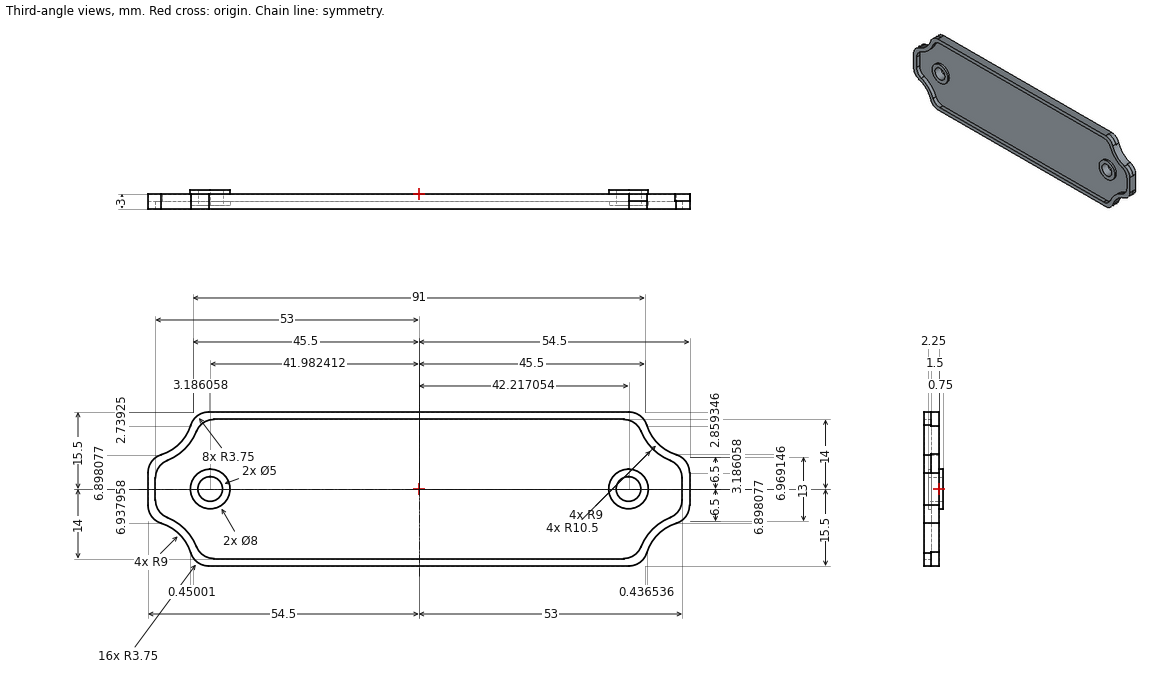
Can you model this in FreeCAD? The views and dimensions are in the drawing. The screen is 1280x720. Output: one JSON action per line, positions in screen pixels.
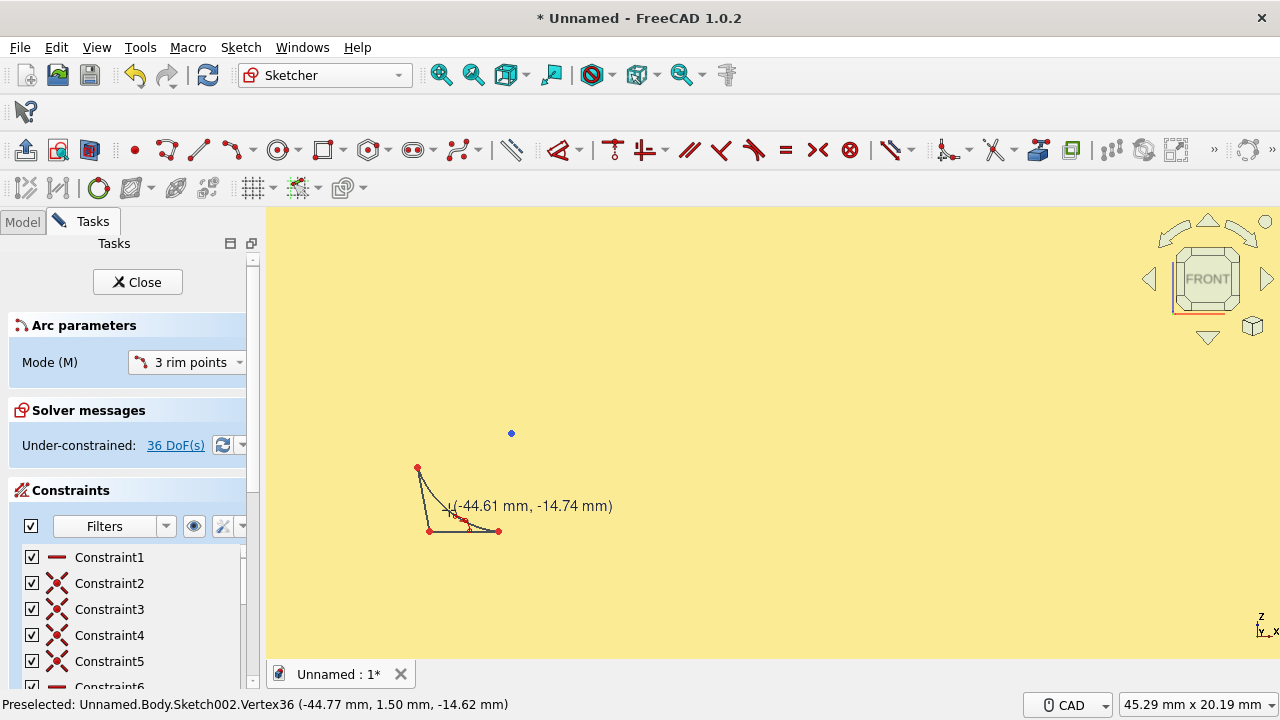
{"action": "left_click", "coordinate": [168, 150]}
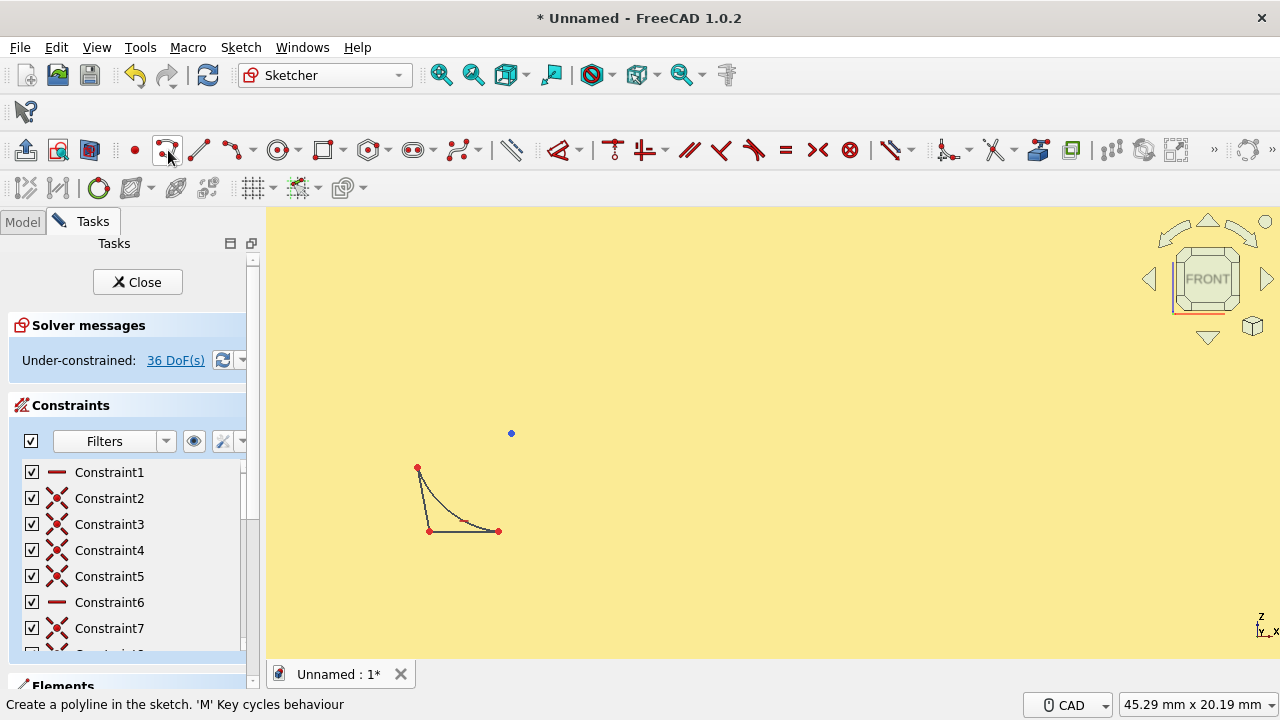
{"action": "scroll", "coordinate": [461, 516], "scroll_direction": "down", "scroll_amount": 7}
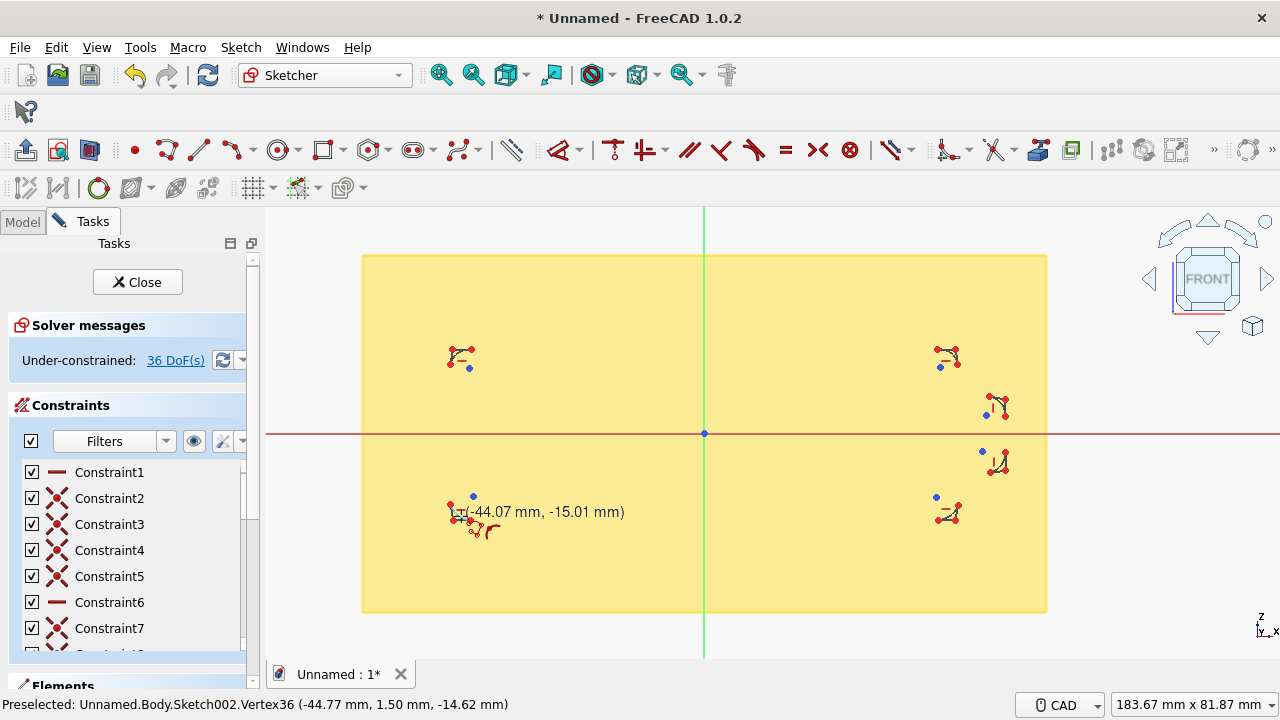
{"action": "left_click", "coordinate": [404, 452]}
{"action": "left_click", "coordinate": [404, 470]}
{"action": "left_click", "coordinate": [419, 472]}
{"action": "right_click", "coordinate": [419, 472]}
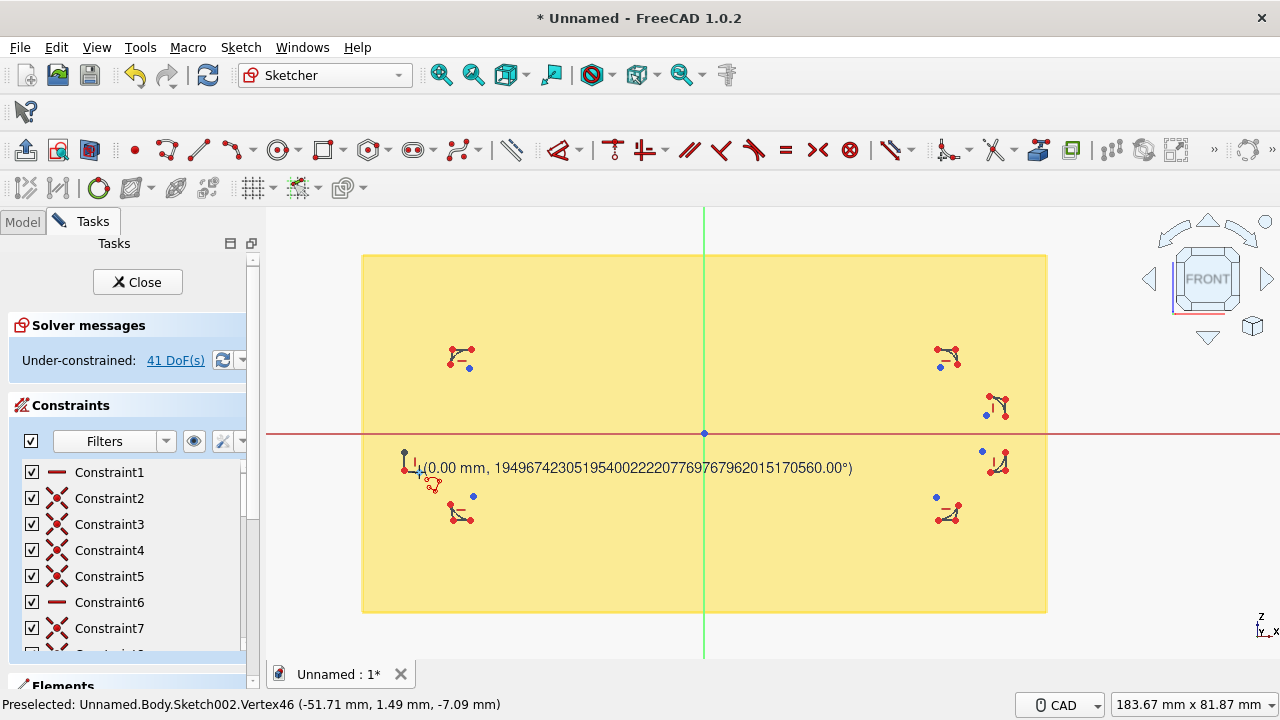
{"action": "left_click", "coordinate": [232, 150]}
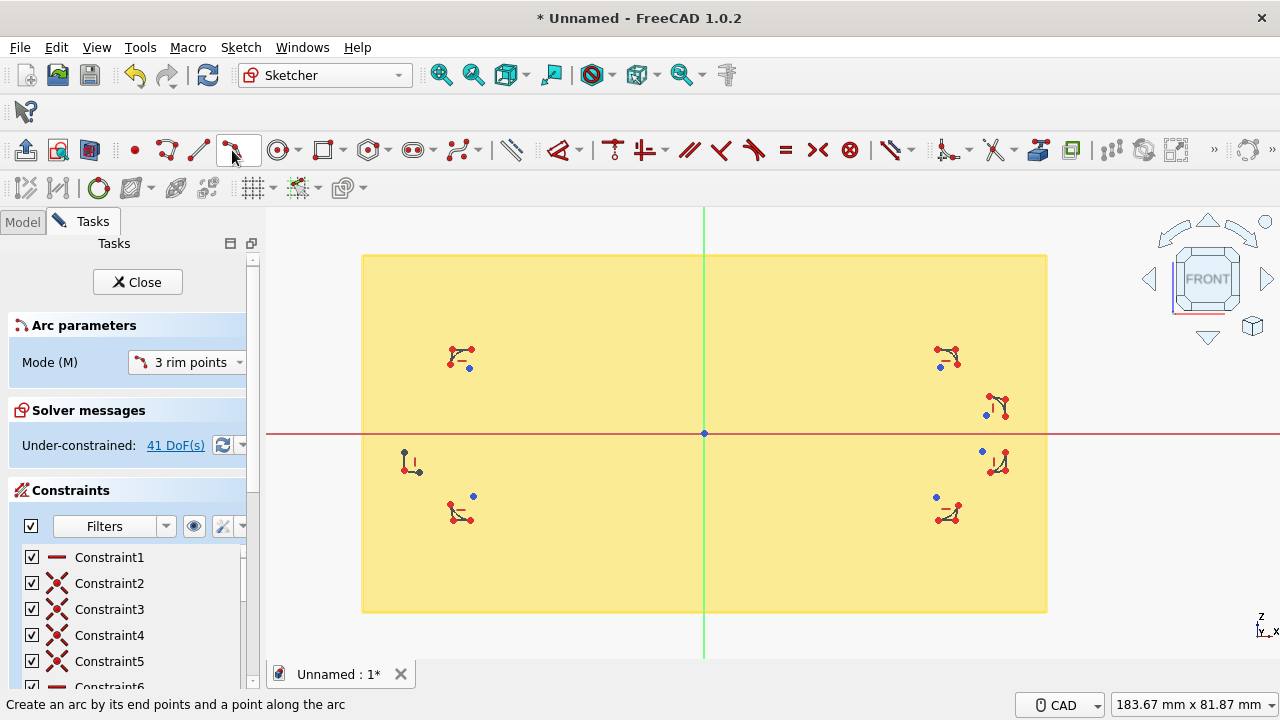
{"action": "scroll", "coordinate": [419, 472], "scroll_direction": "up", "scroll_amount": 4}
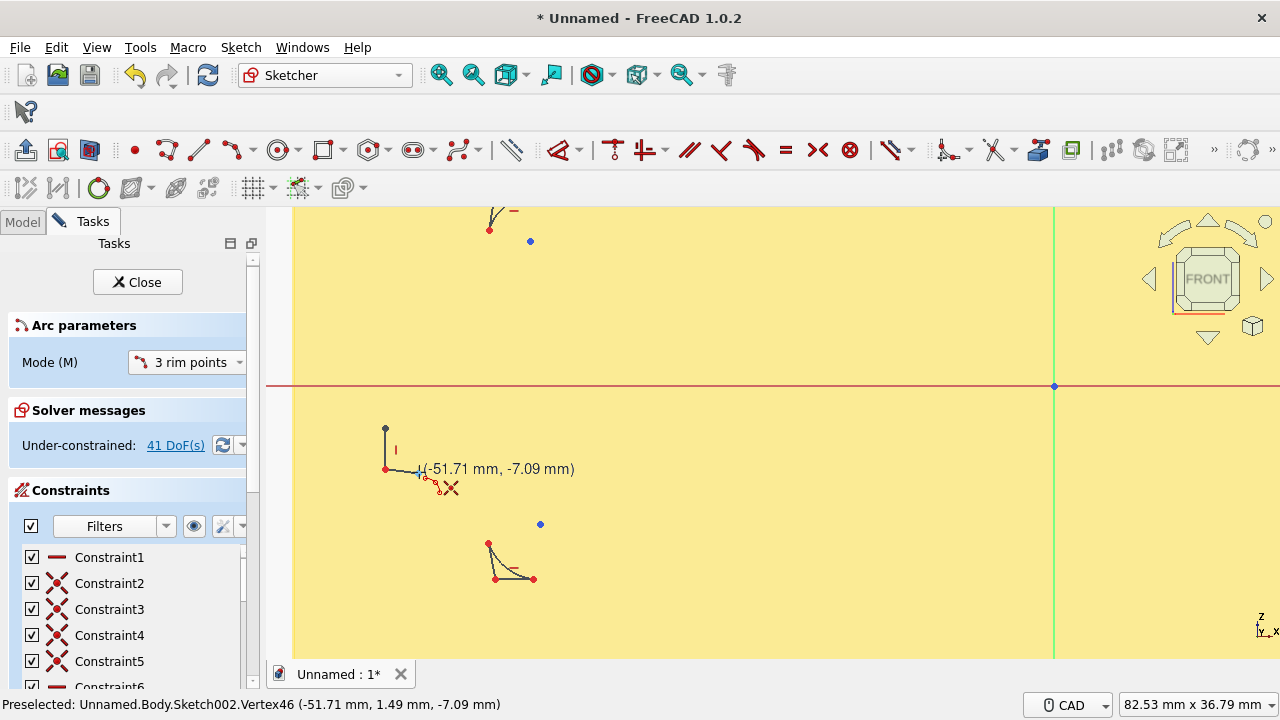
{"action": "left_click", "coordinate": [419, 474]}
{"action": "left_click", "coordinate": [385, 429]}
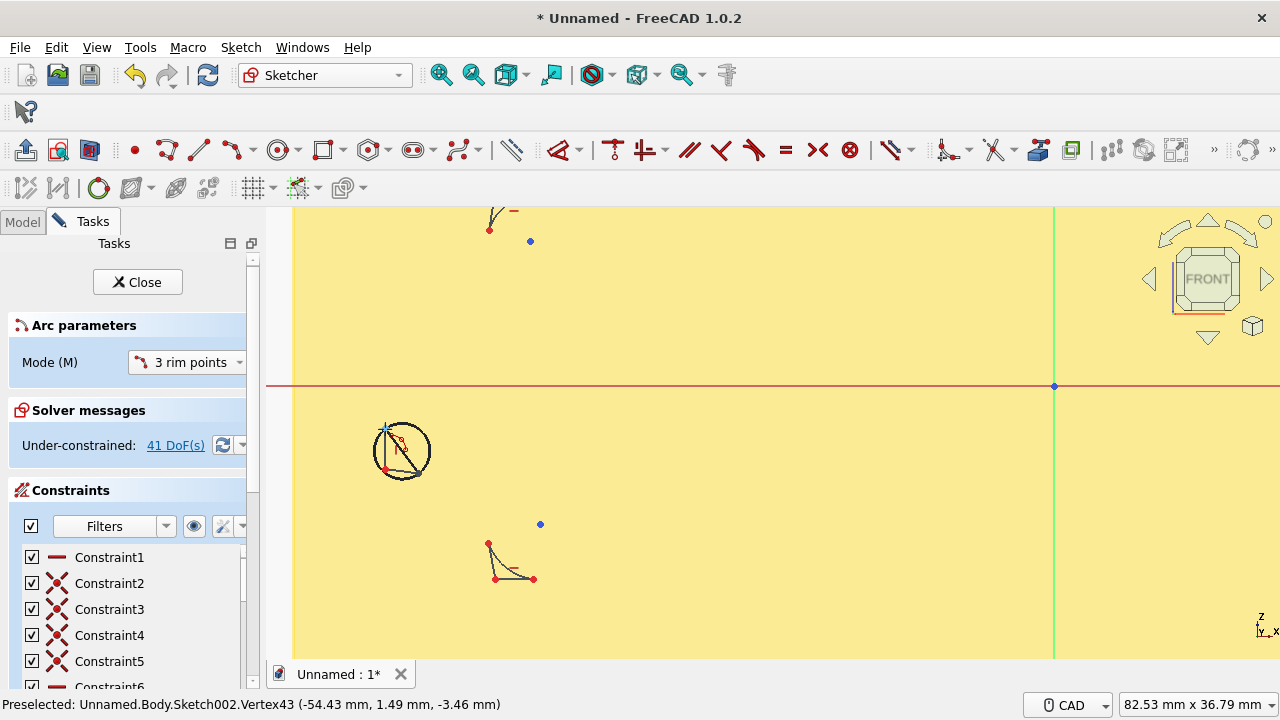
{"action": "scroll", "coordinate": [394, 455], "scroll_direction": "up", "scroll_amount": 3}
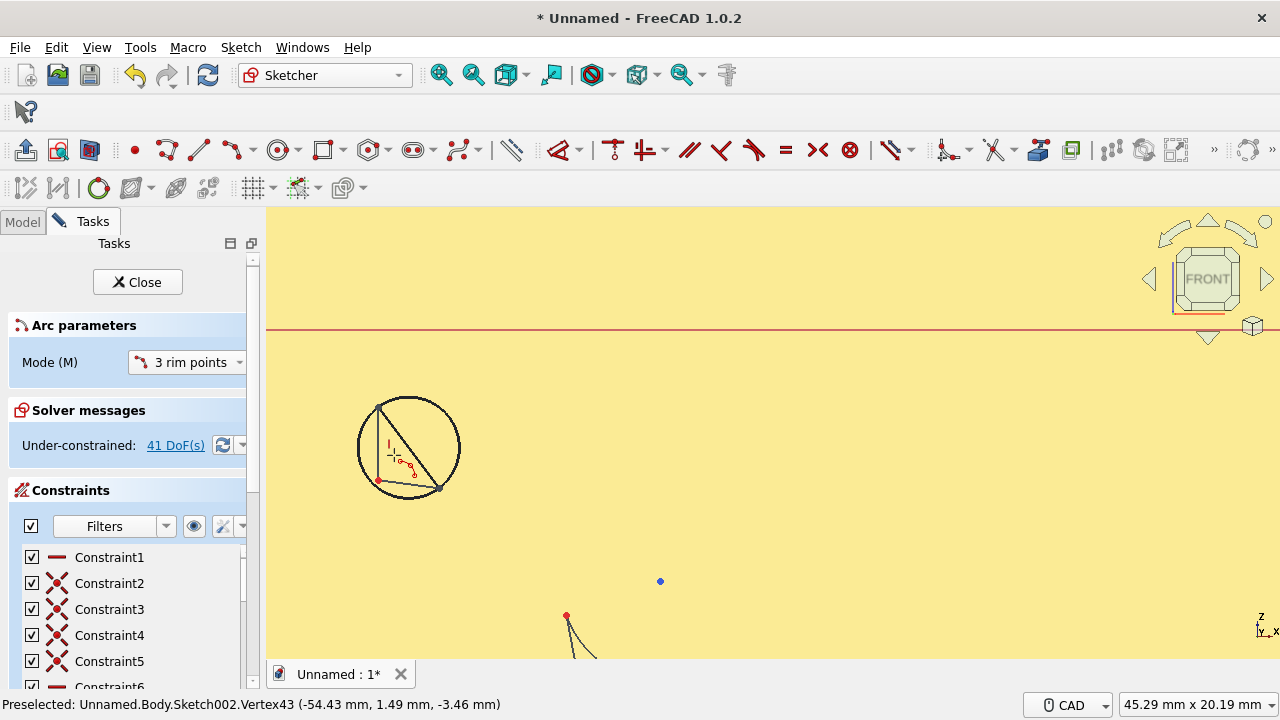
{"action": "left_click", "coordinate": [394, 455]}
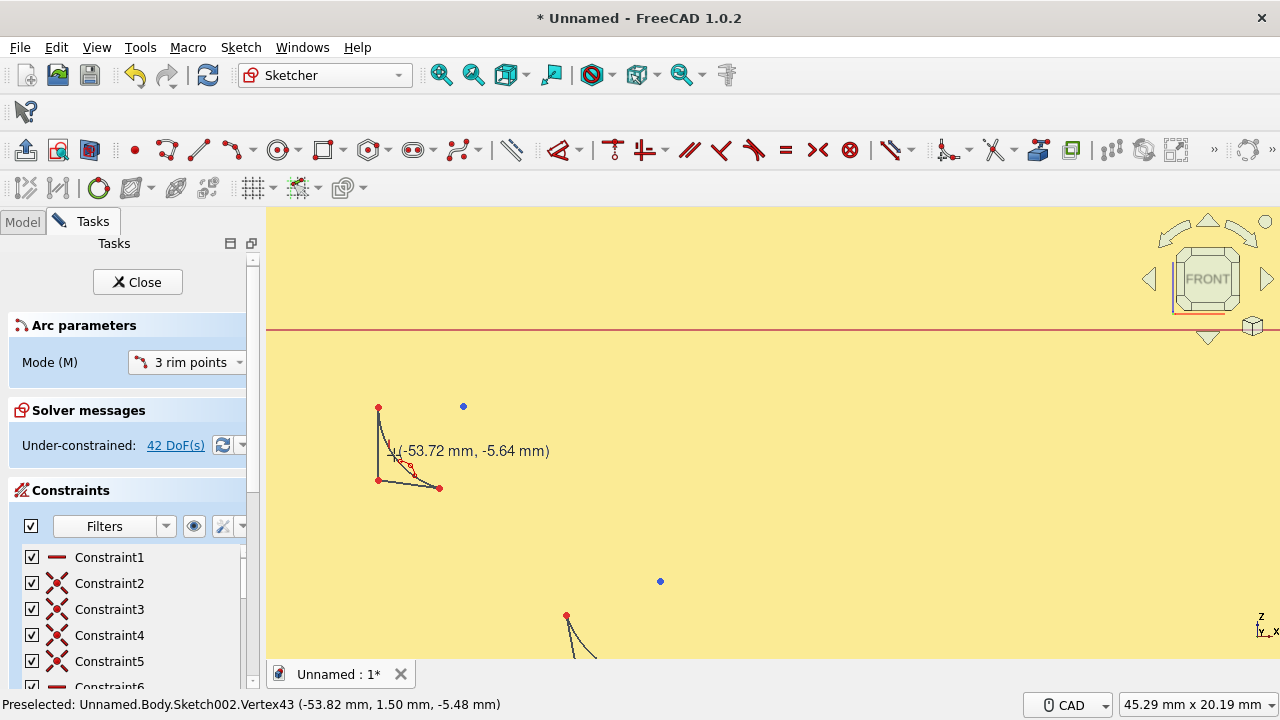
{"action": "left_click", "coordinate": [168, 150]}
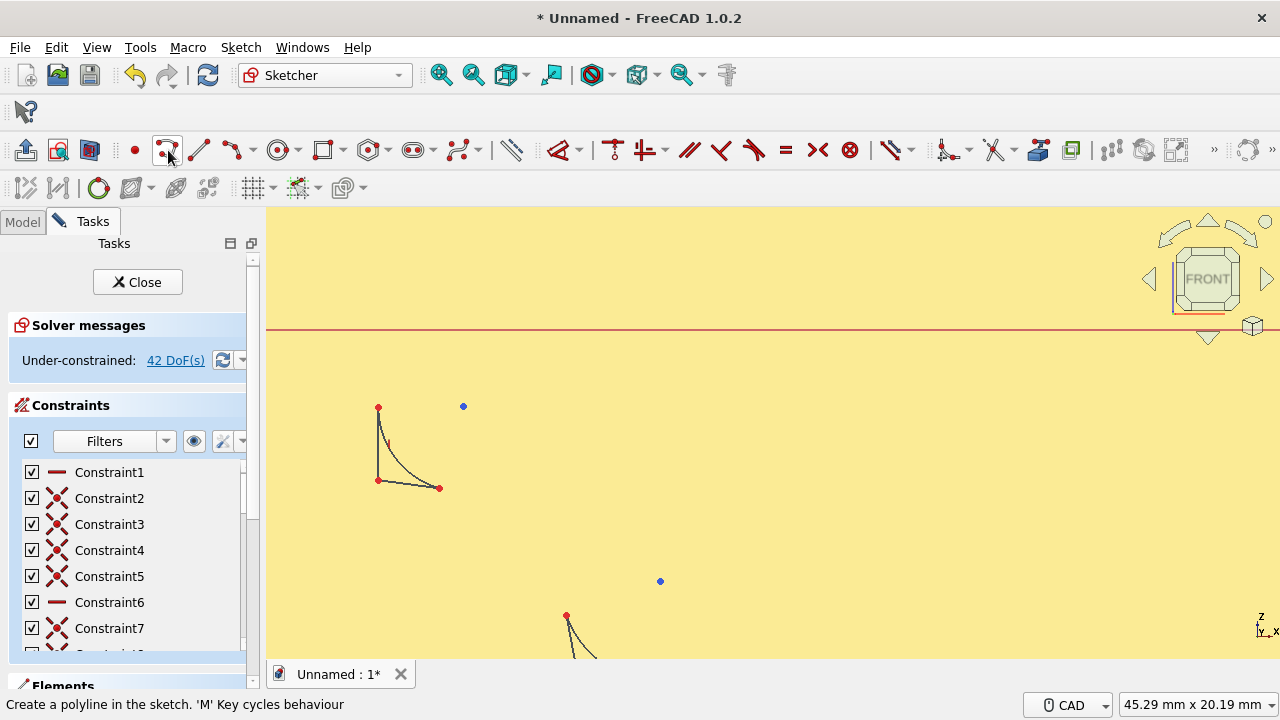
{"action": "scroll", "coordinate": [412, 467], "scroll_direction": "down", "scroll_amount": 7}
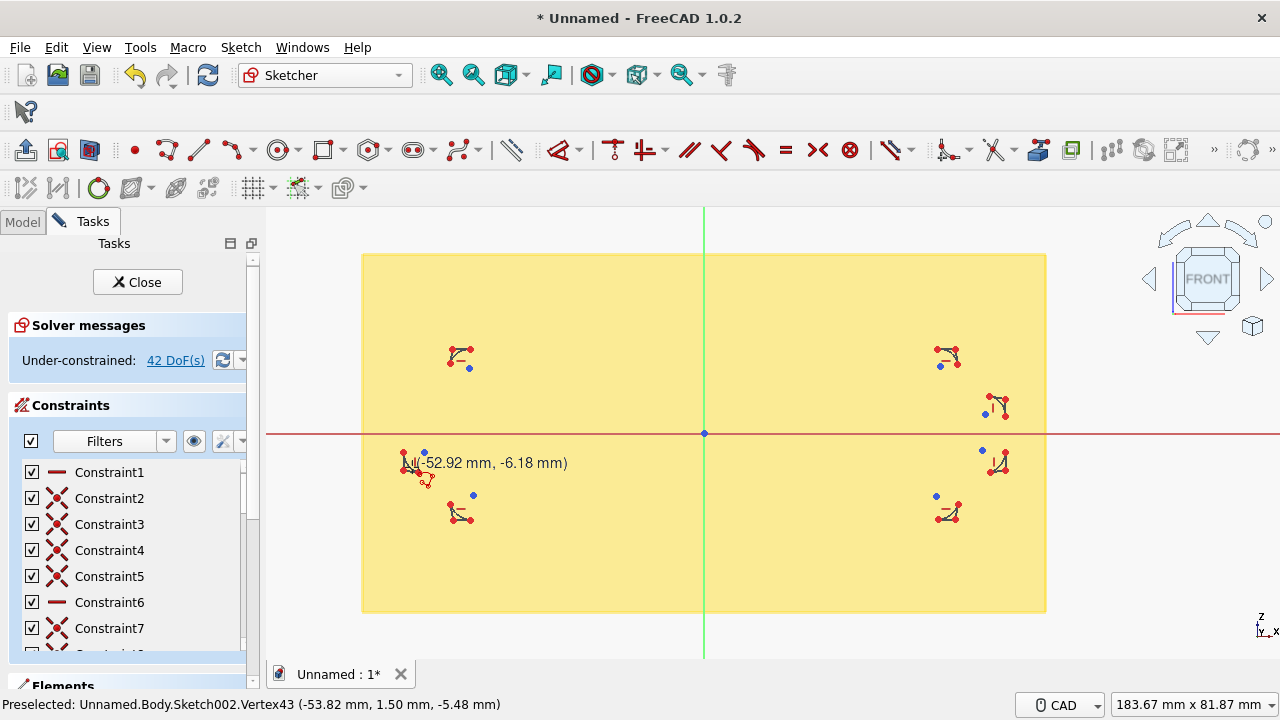
{"action": "left_click", "coordinate": [418, 395]}
{"action": "left_click", "coordinate": [403, 398]}
{"action": "left_click", "coordinate": [403, 415]}
{"action": "right_click", "coordinate": [403, 415]}